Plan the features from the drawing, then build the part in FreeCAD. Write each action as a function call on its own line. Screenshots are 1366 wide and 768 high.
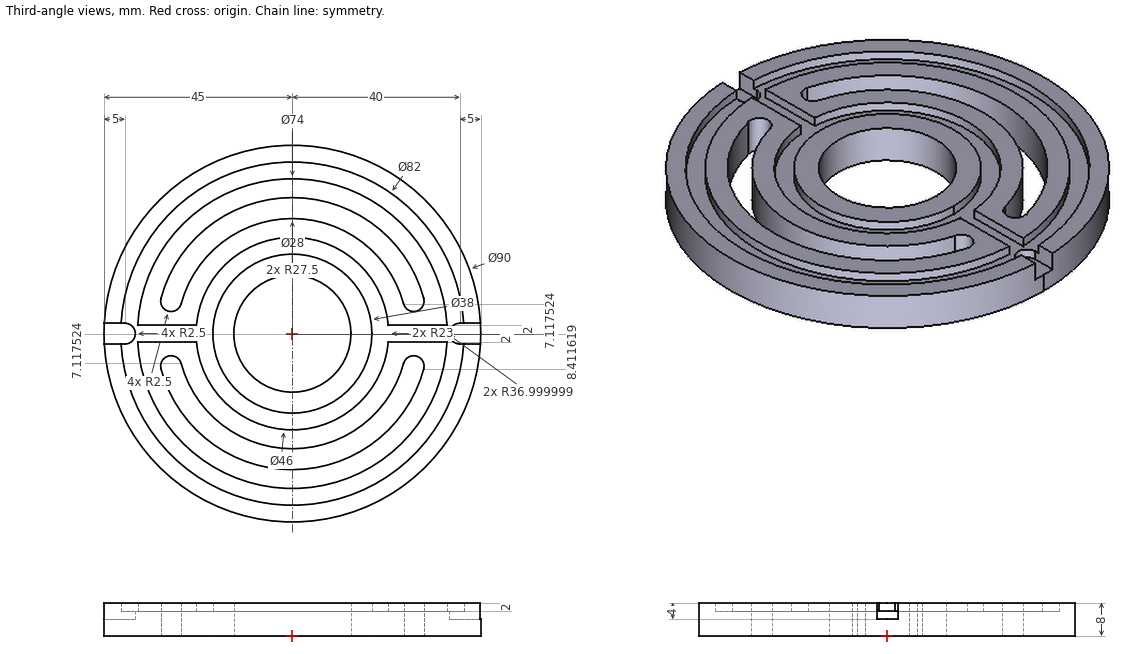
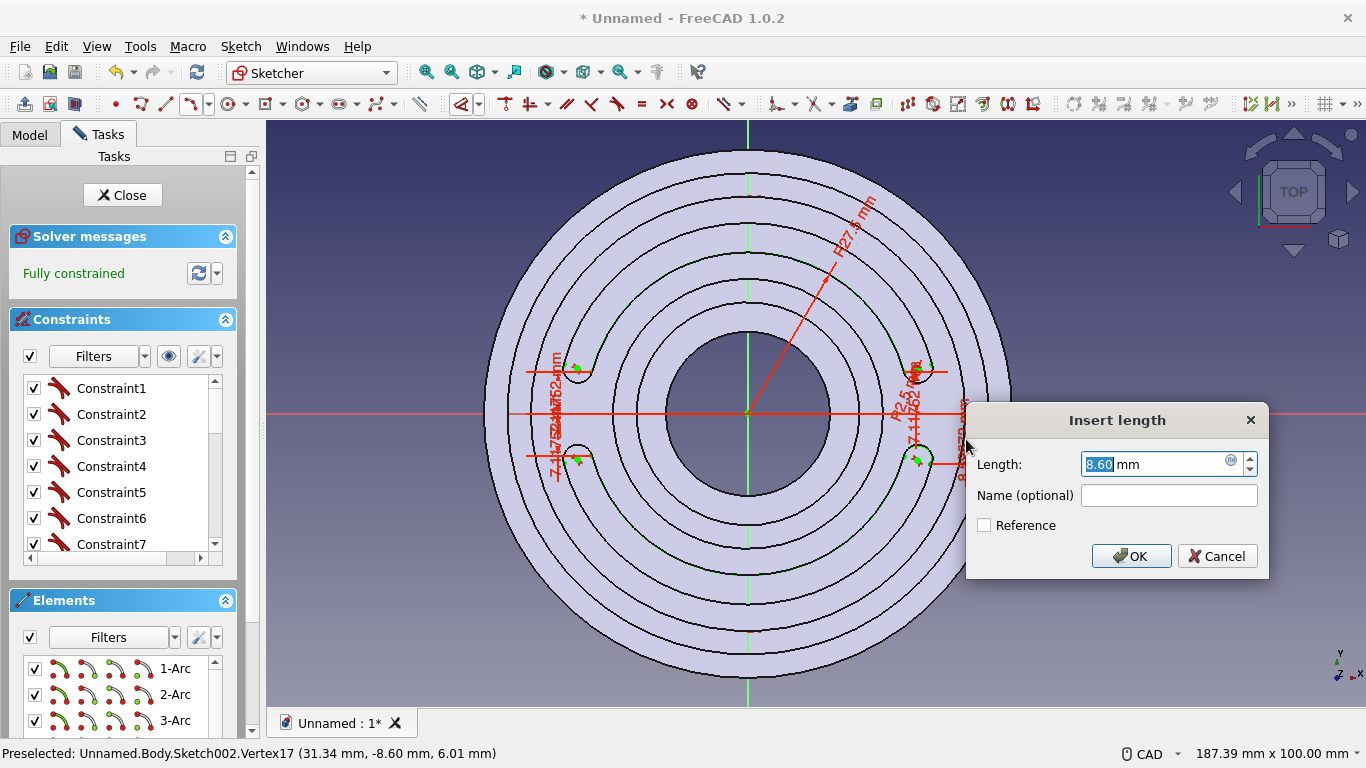
text(8.411619)
key(Return)
key(Escape)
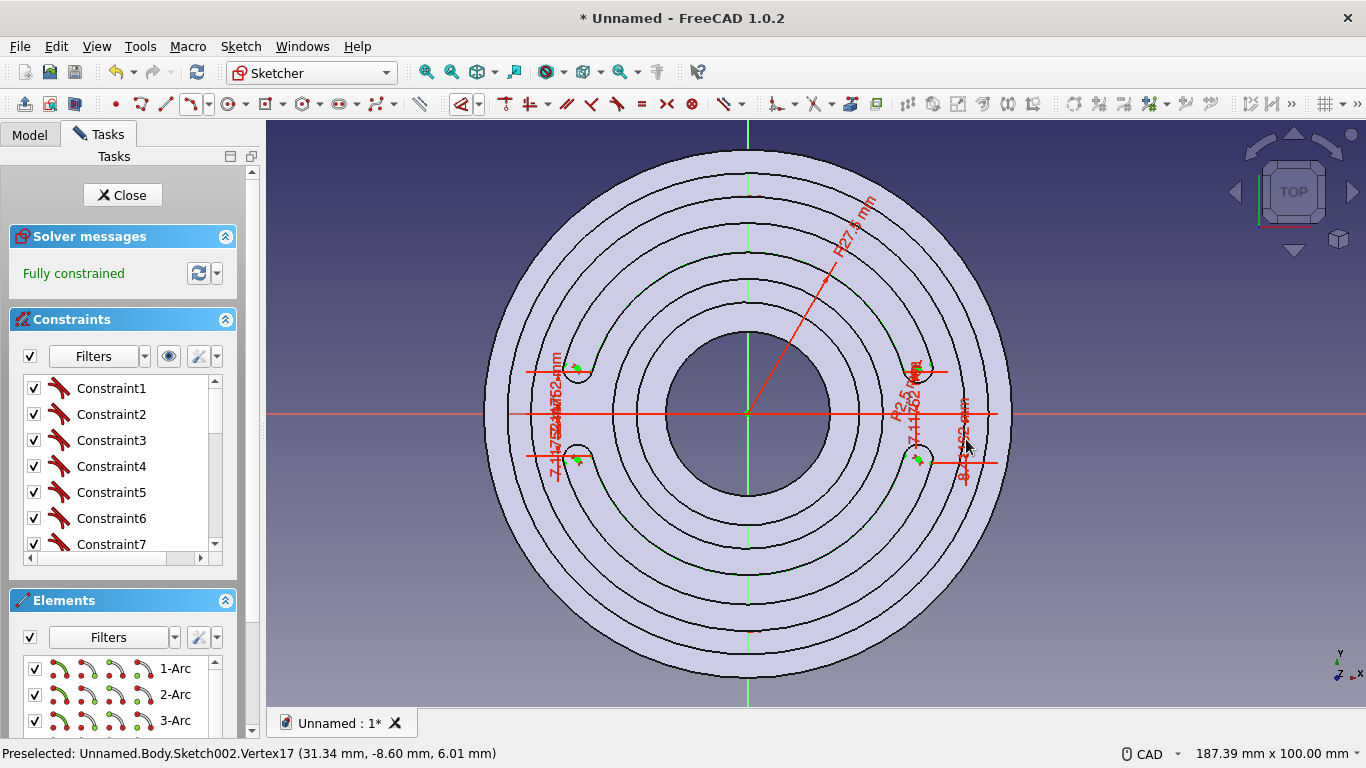
click(123, 195)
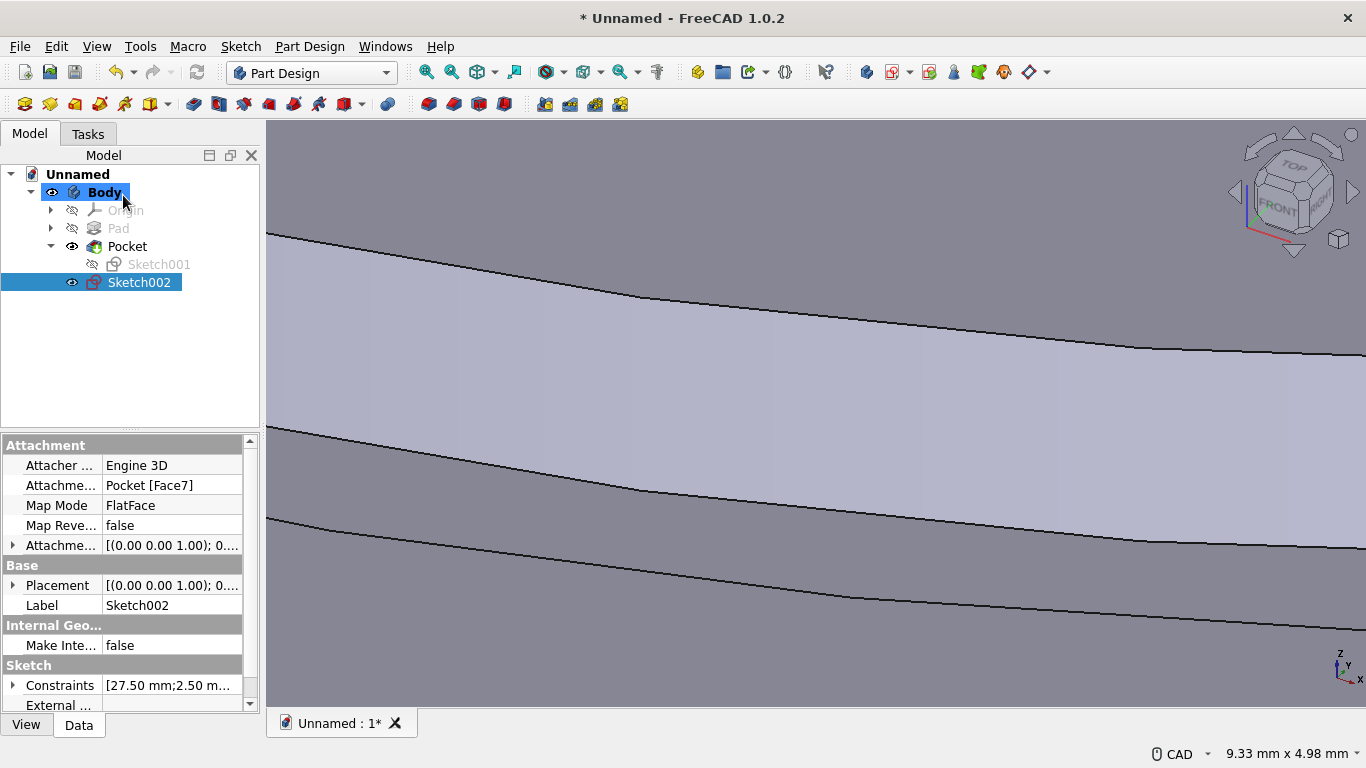
click(194, 104)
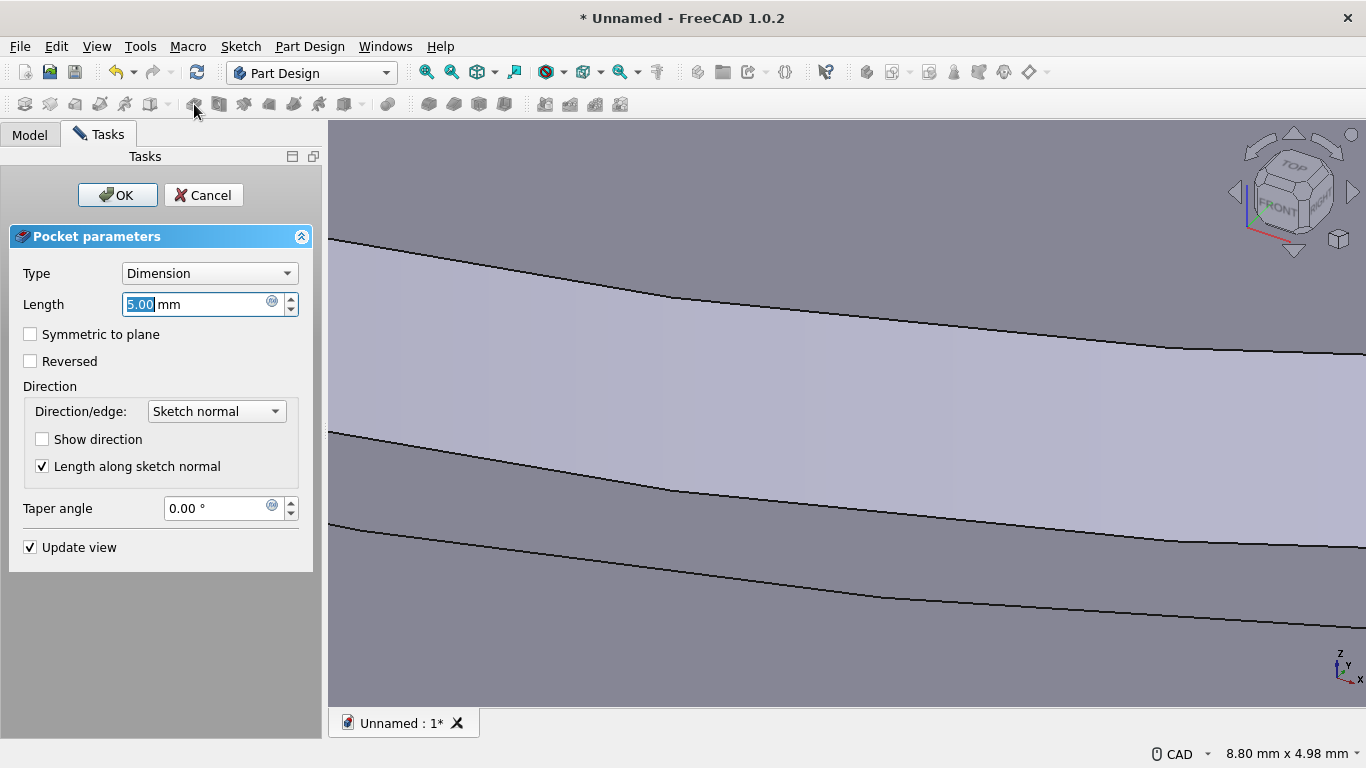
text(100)
key(Tab)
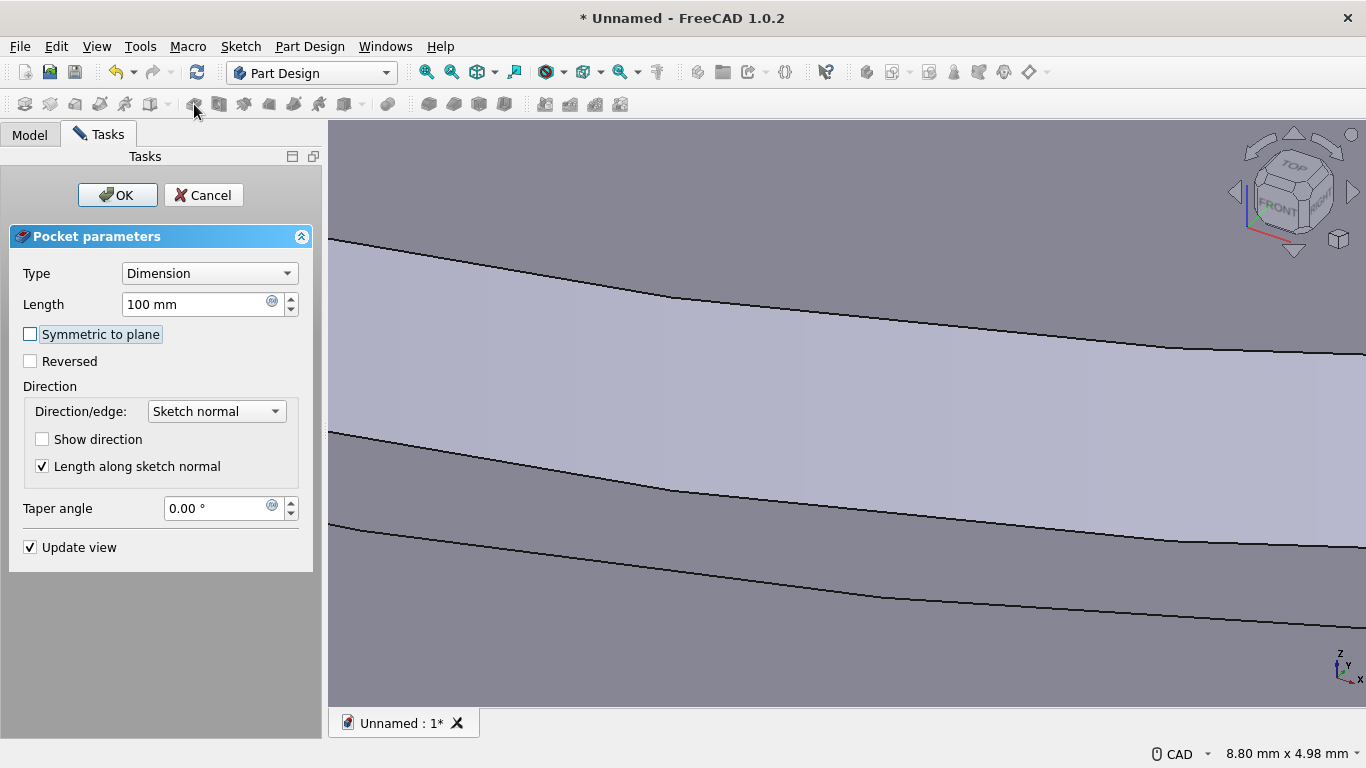
click(118, 195)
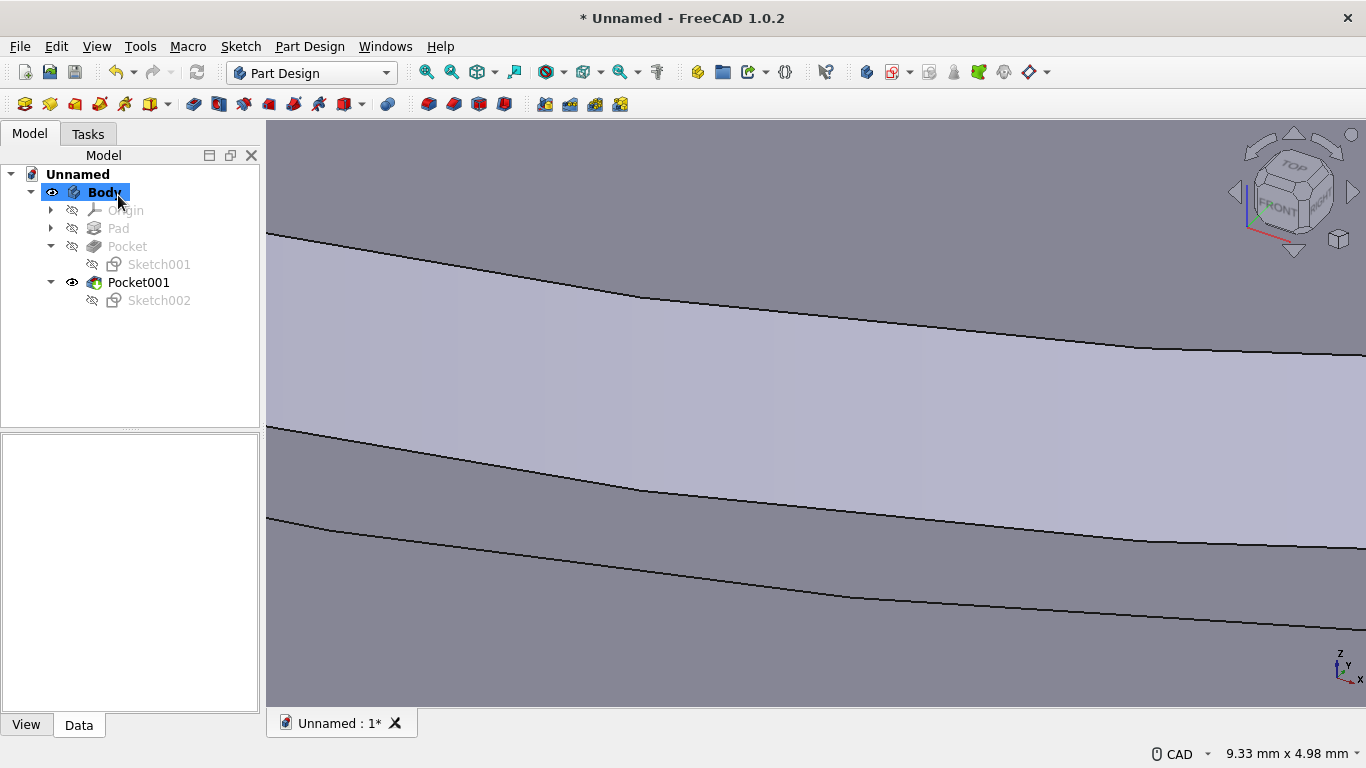
key(v)
key(f)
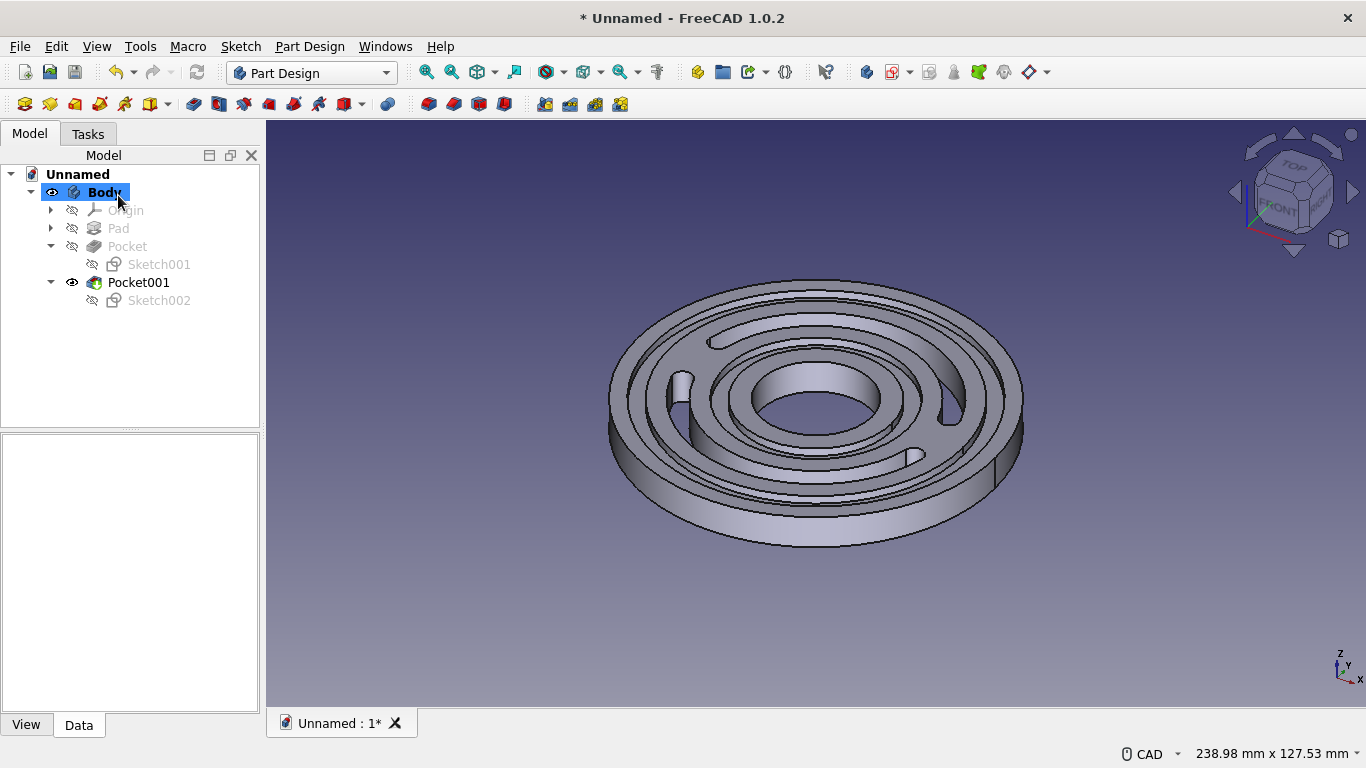
click(942, 439)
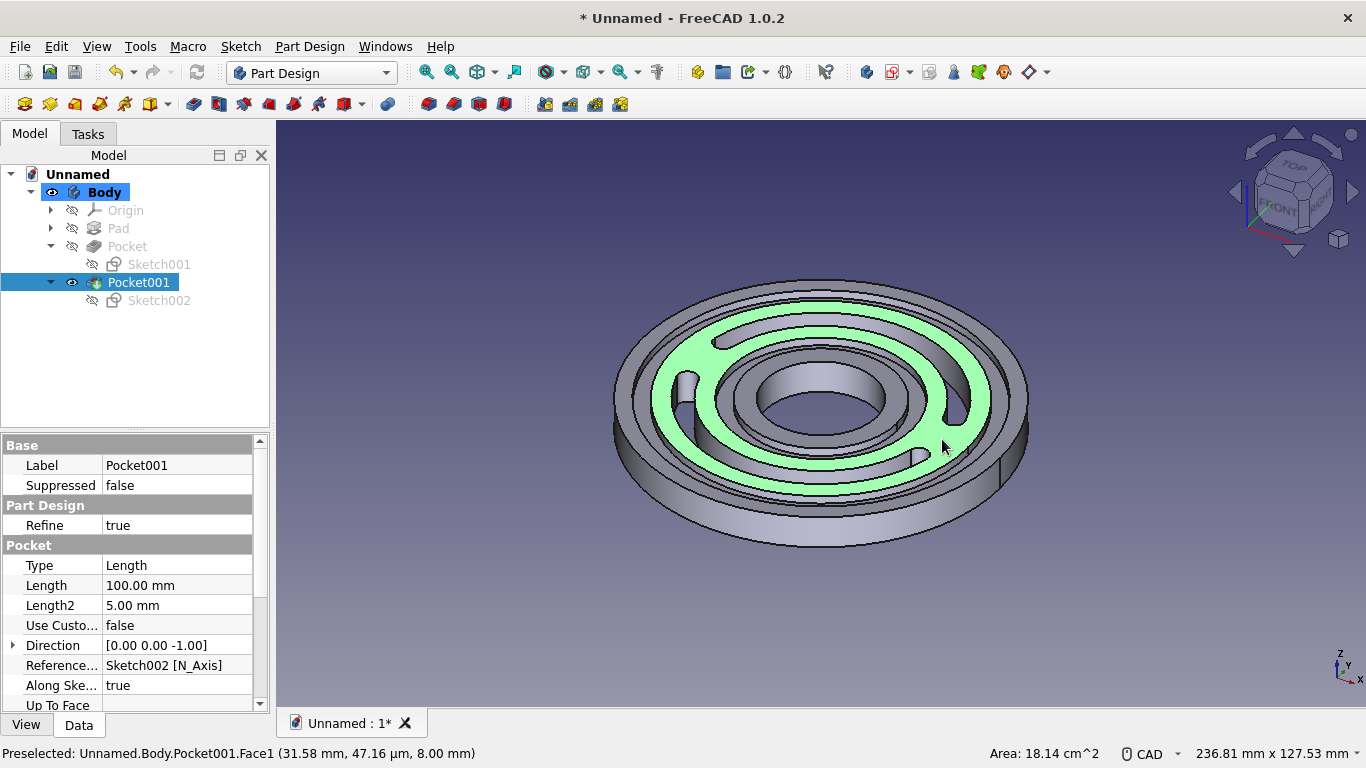
click(892, 72)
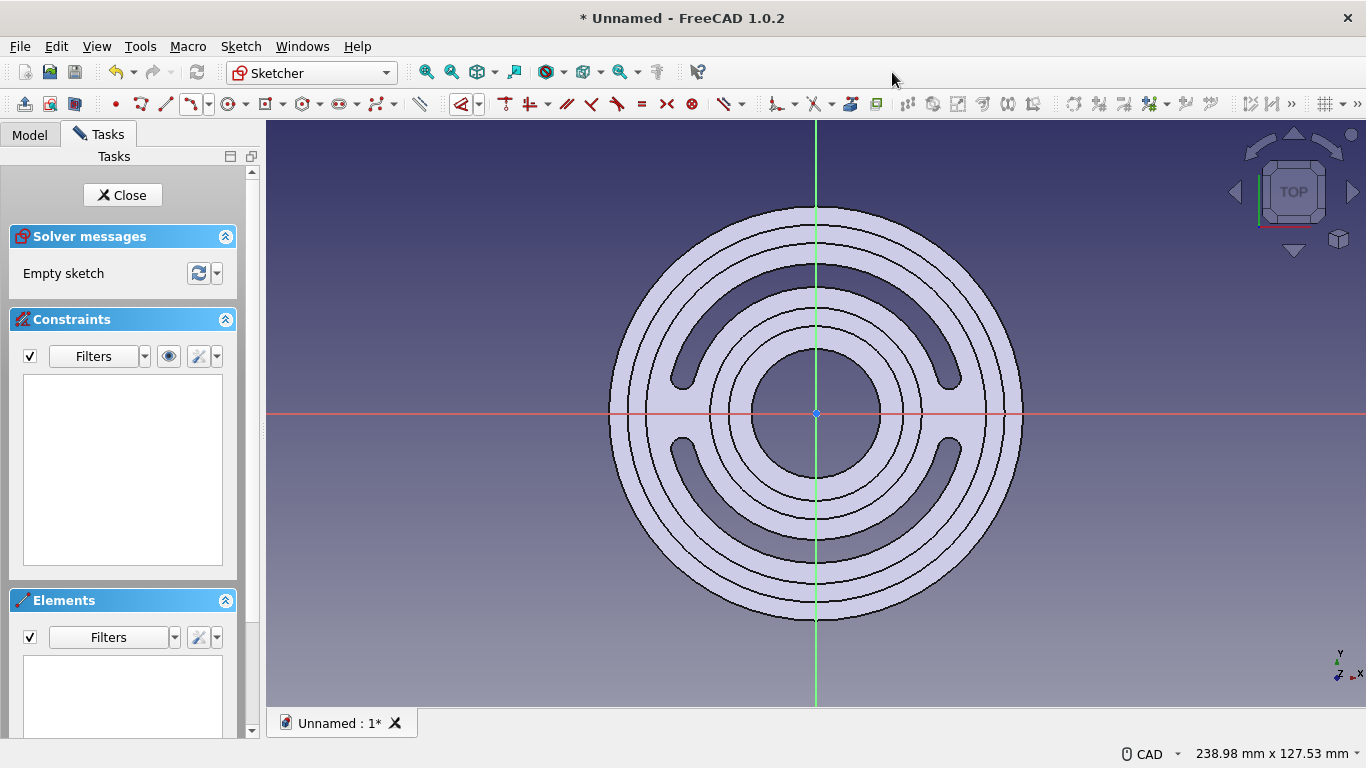
scroll(955, 413, up, 2)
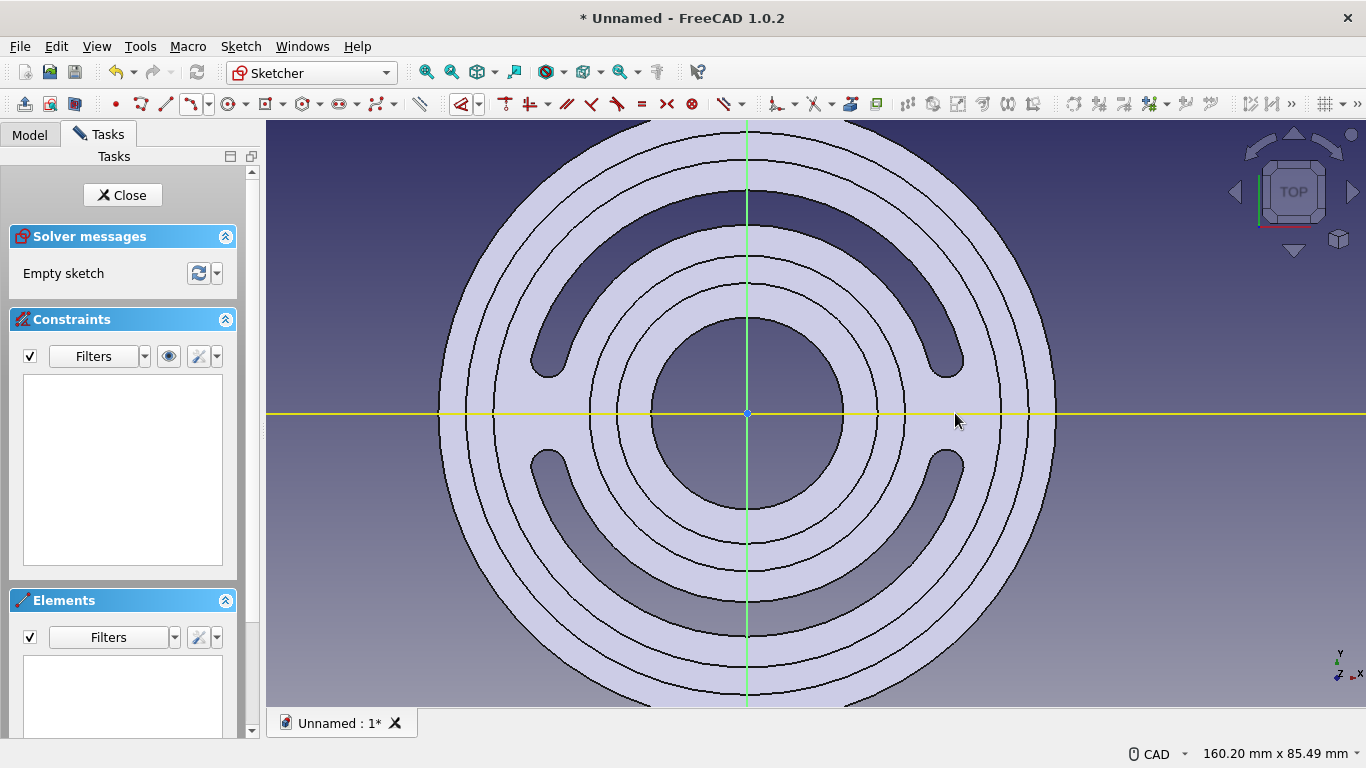
key(g)
key(s)